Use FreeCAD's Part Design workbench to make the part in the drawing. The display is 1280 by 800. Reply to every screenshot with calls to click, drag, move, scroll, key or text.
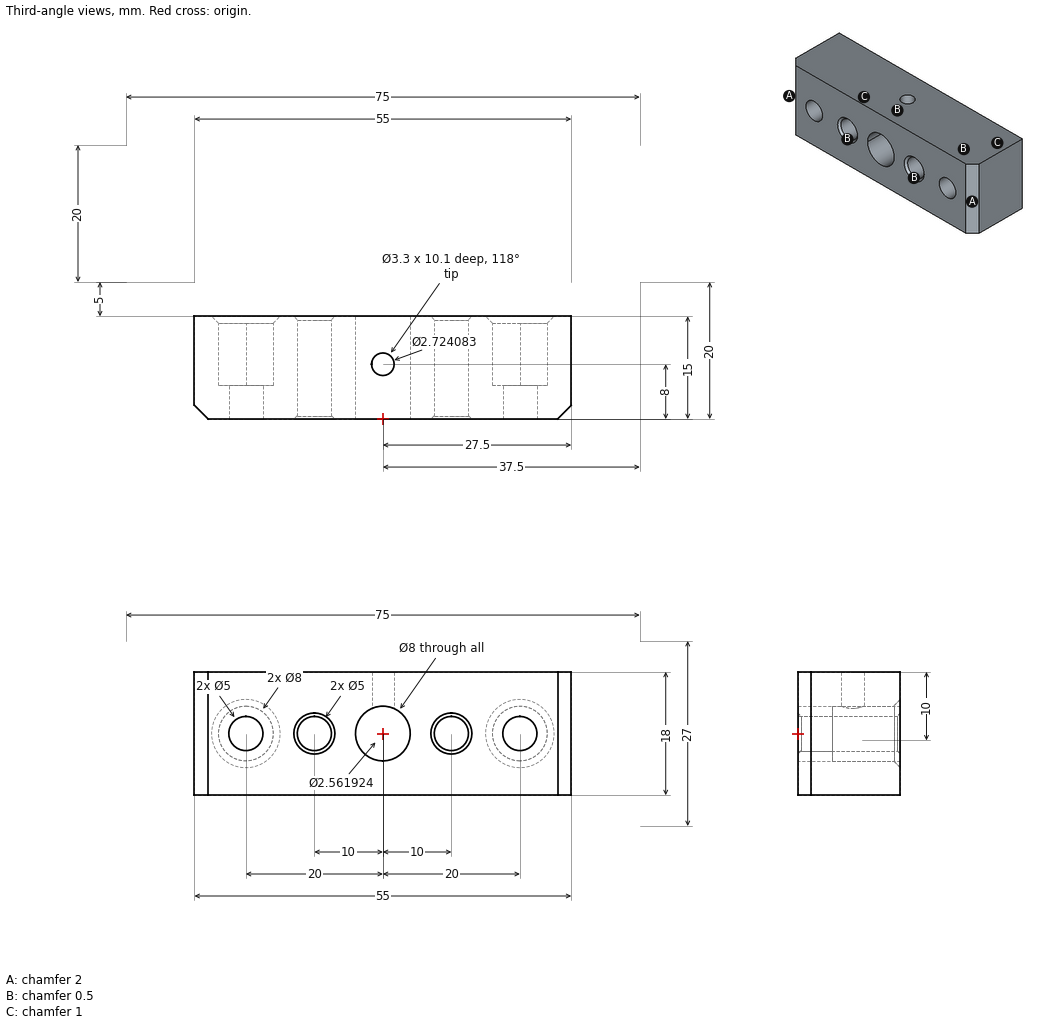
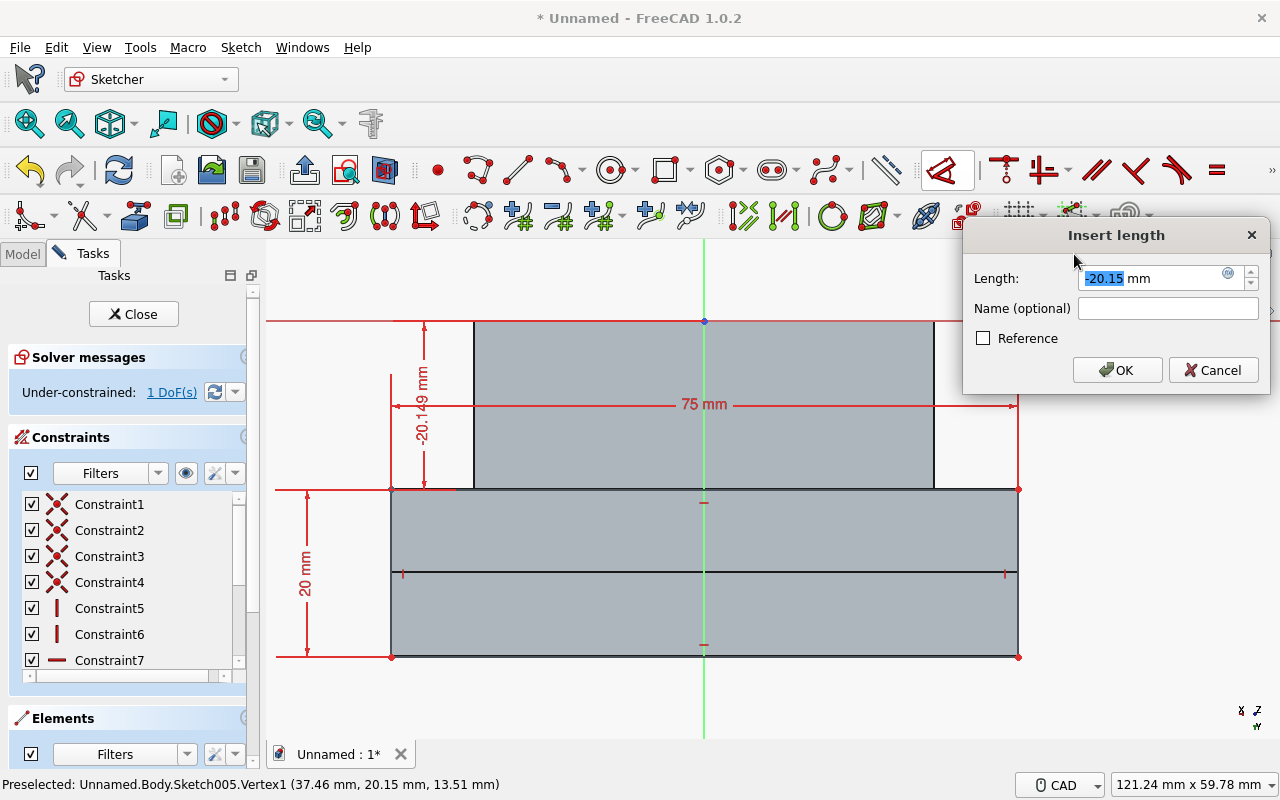
text(-20)
key(Return)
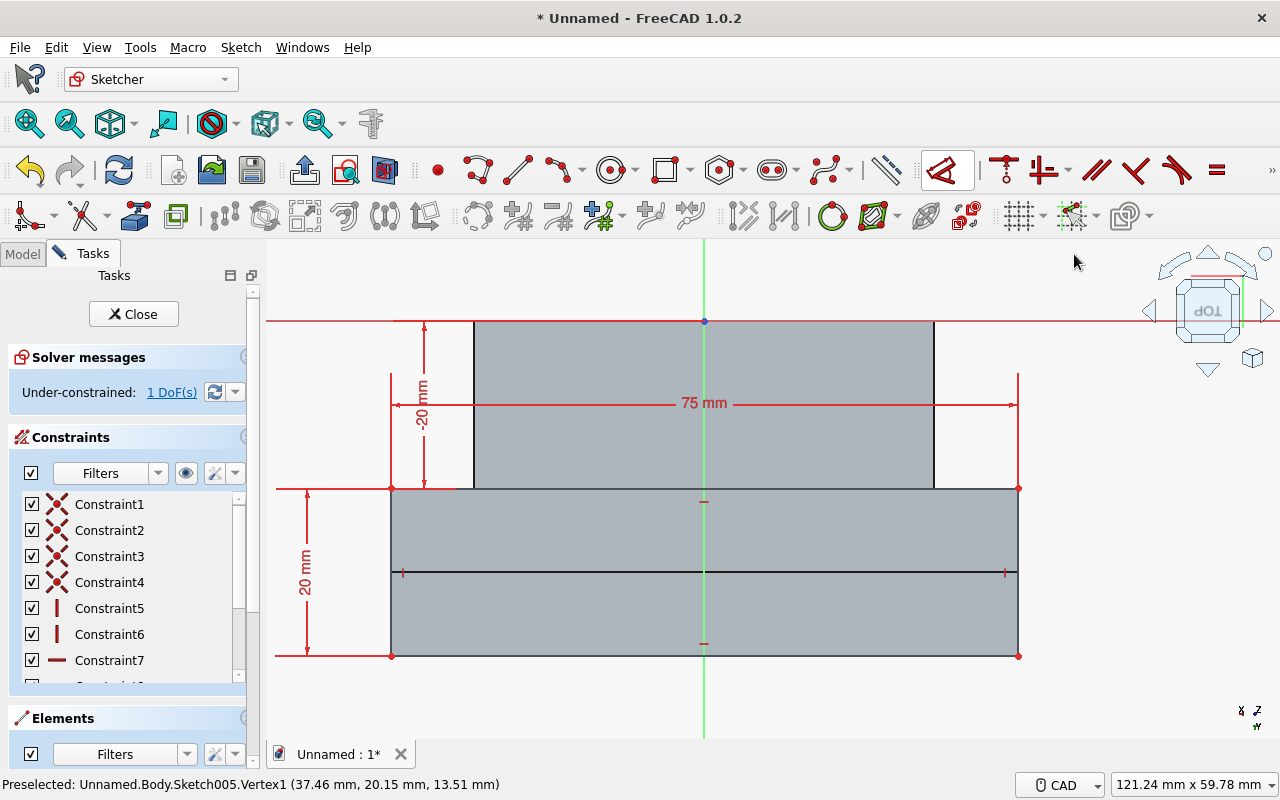
click(391, 489)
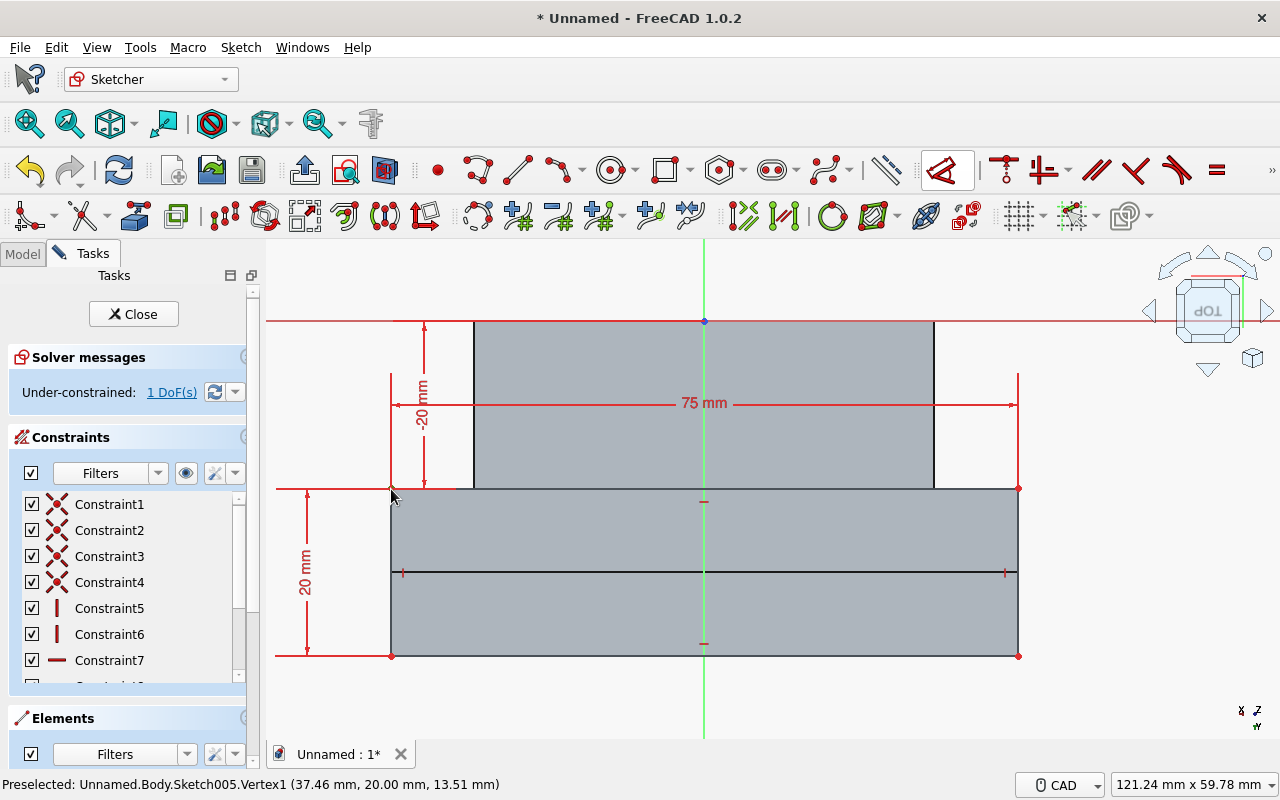
click(968, 170)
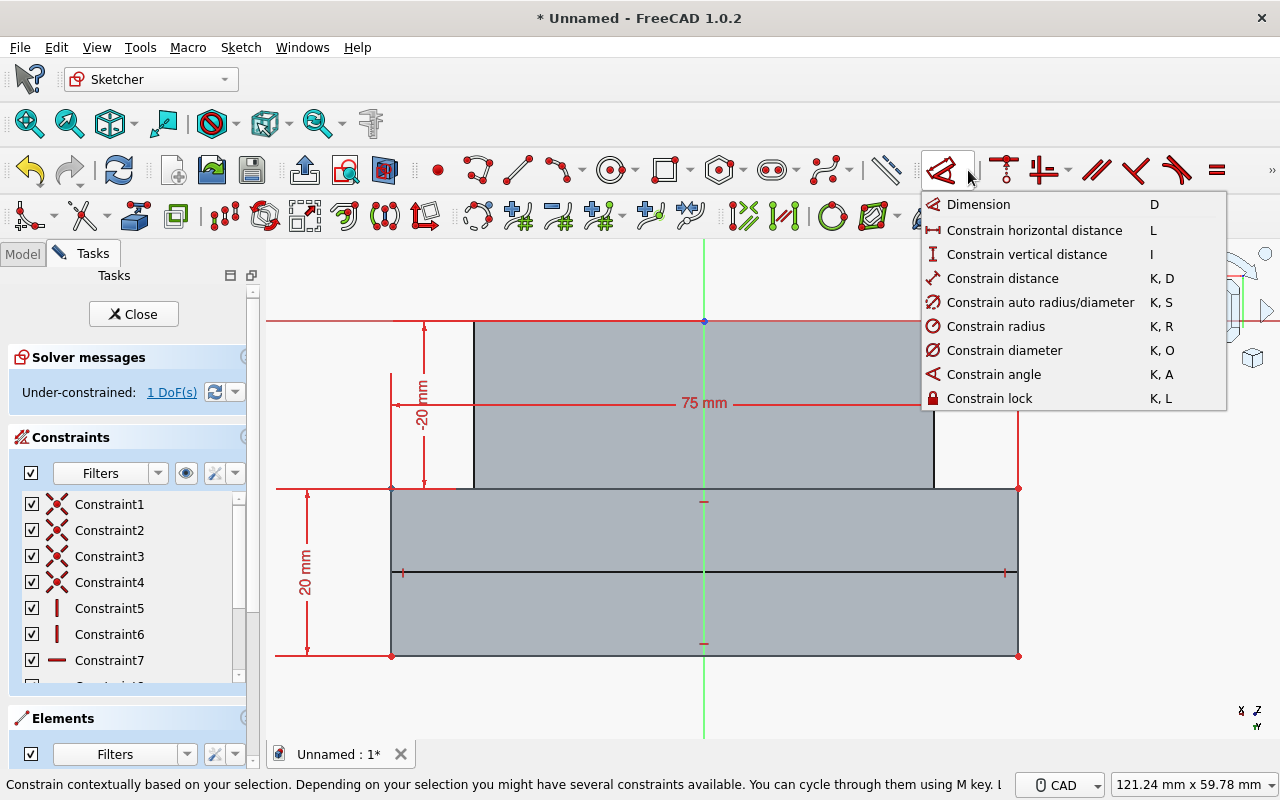
click(1074, 230)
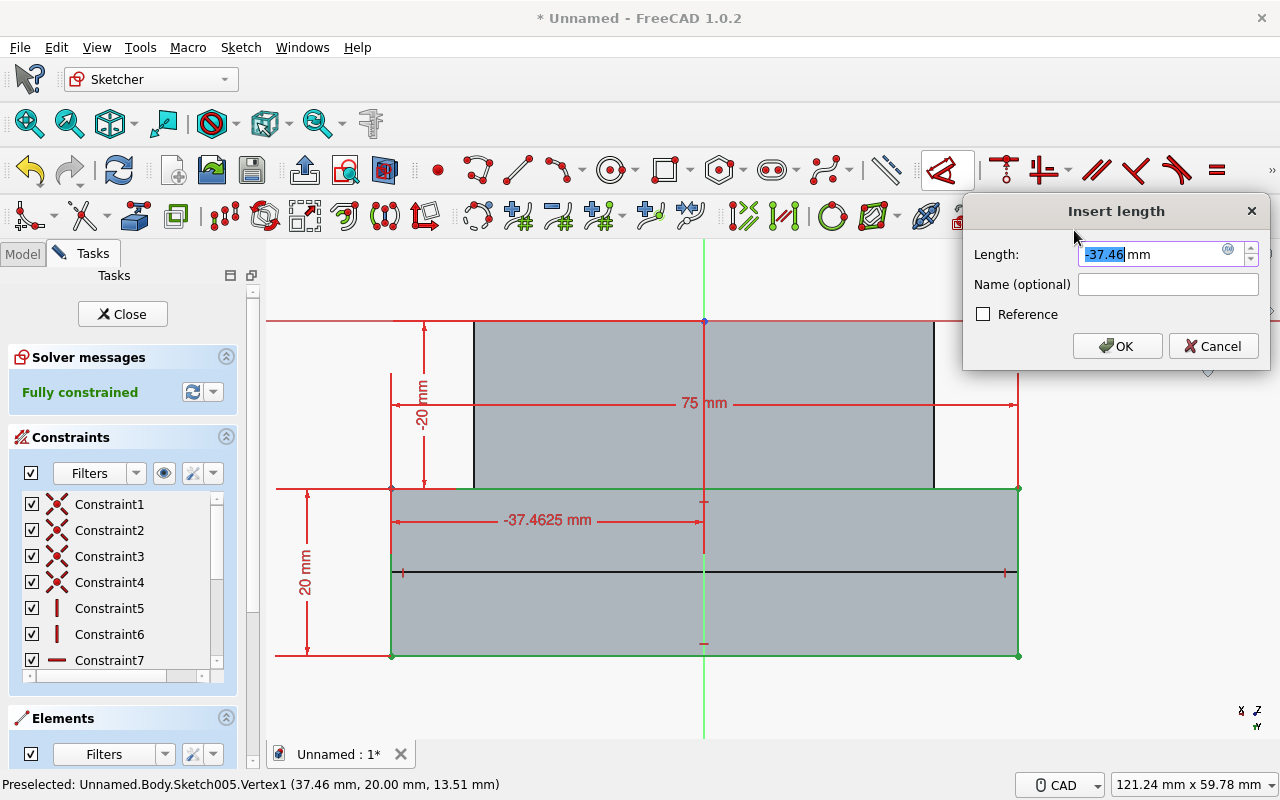
text(-37.5)
key(Return)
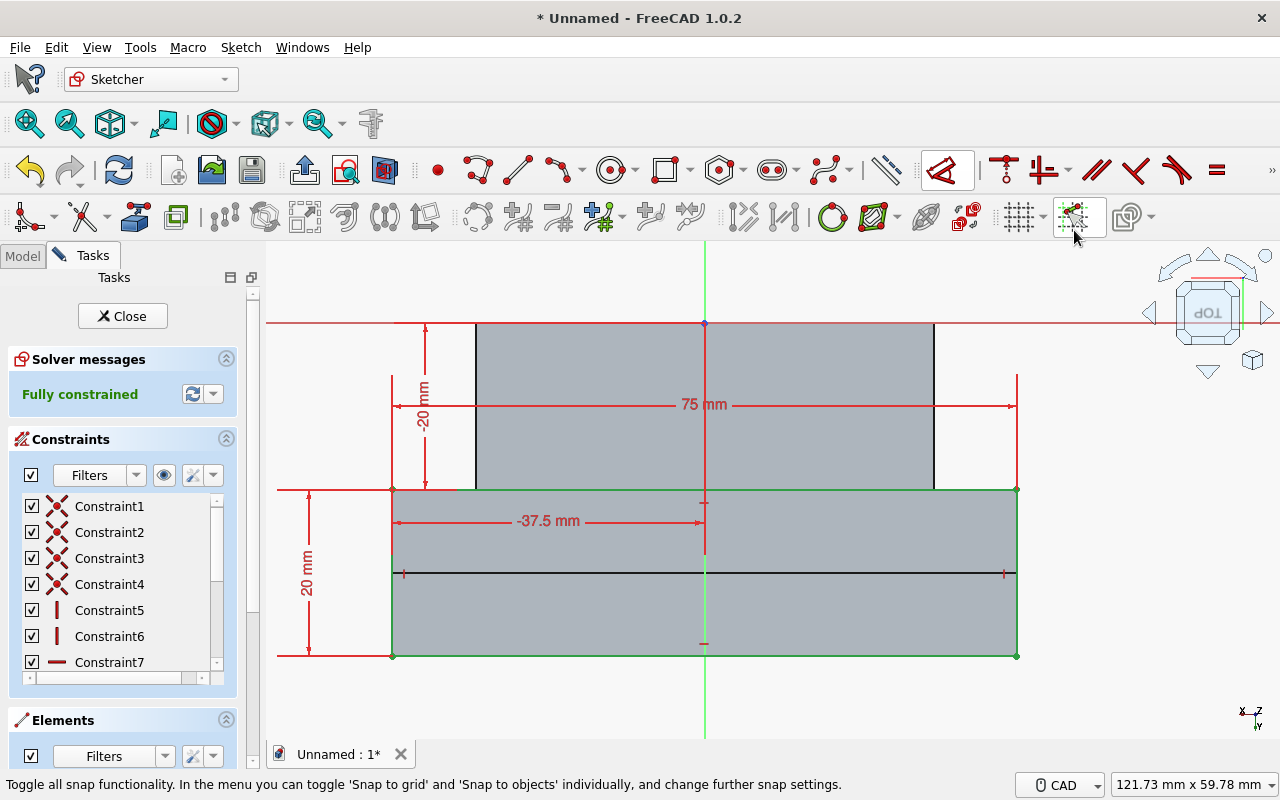
click(123, 316)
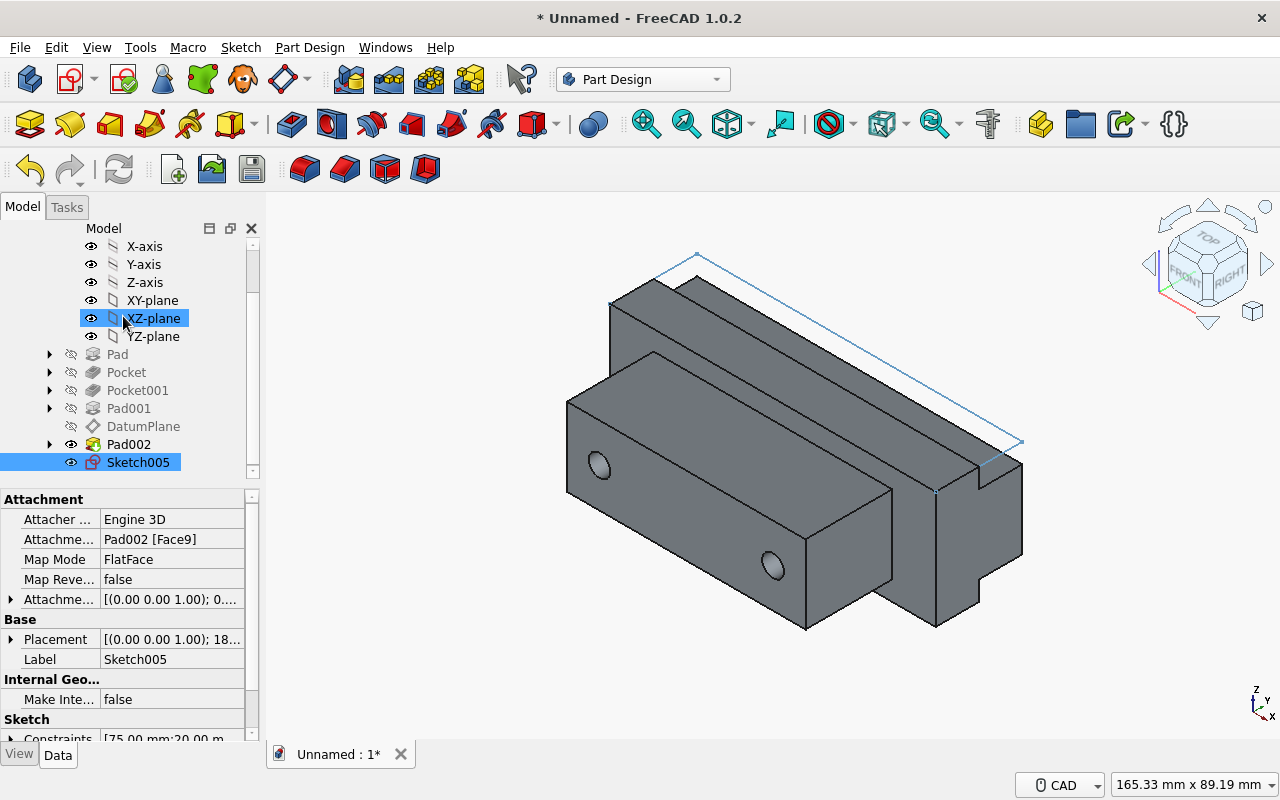
click(292, 124)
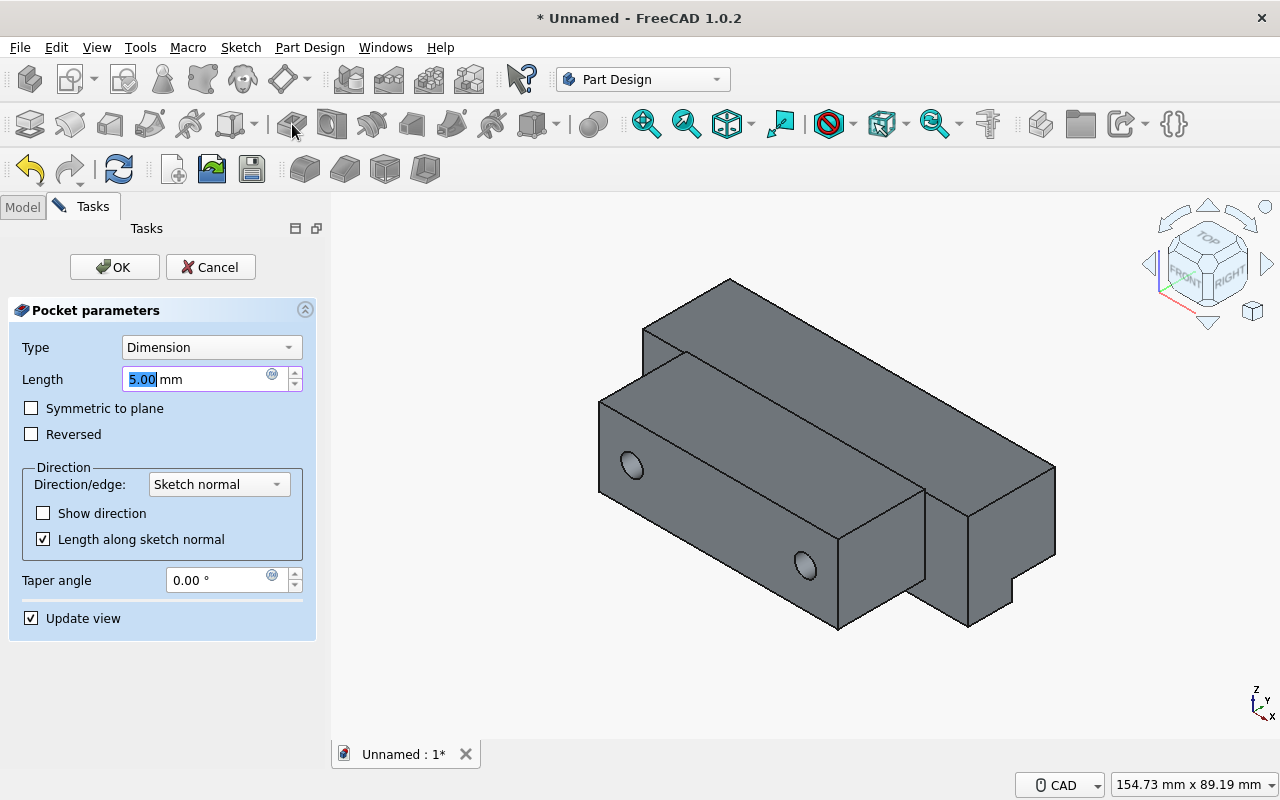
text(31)
key(Tab)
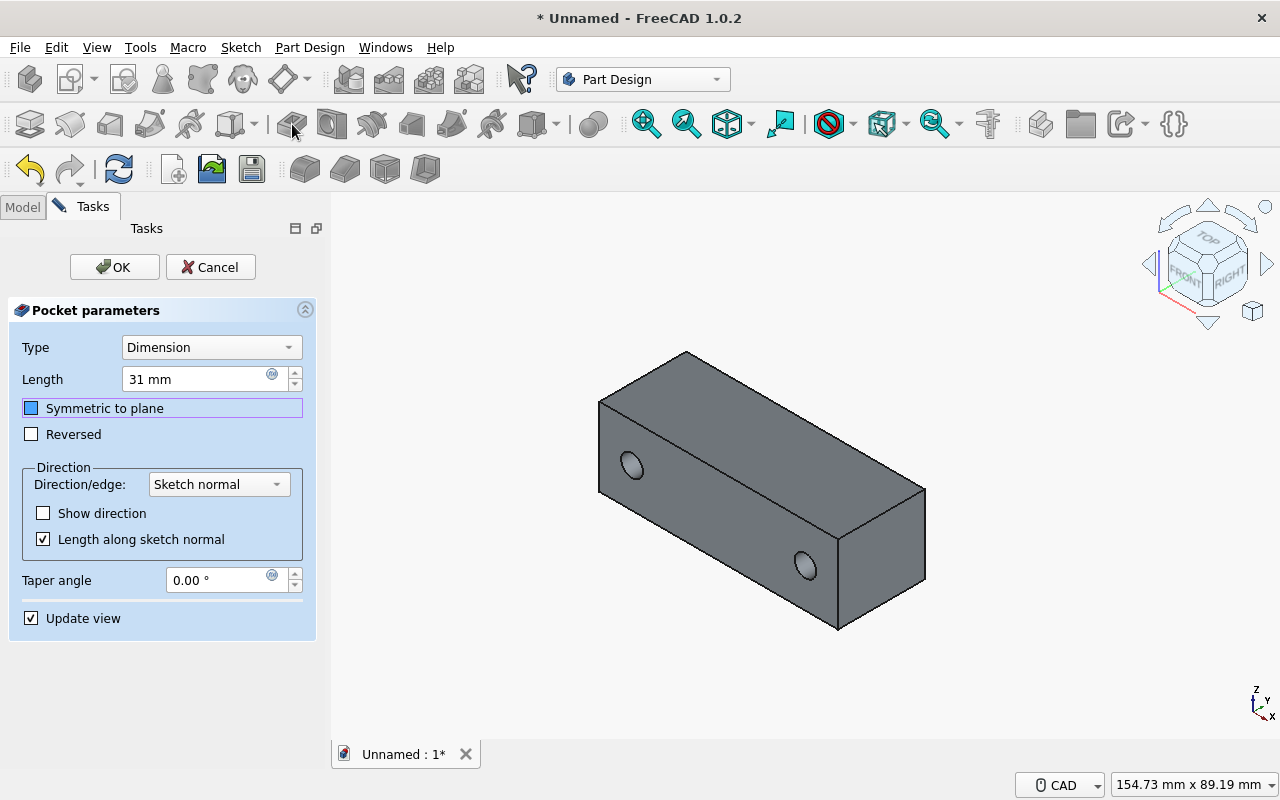
click(115, 267)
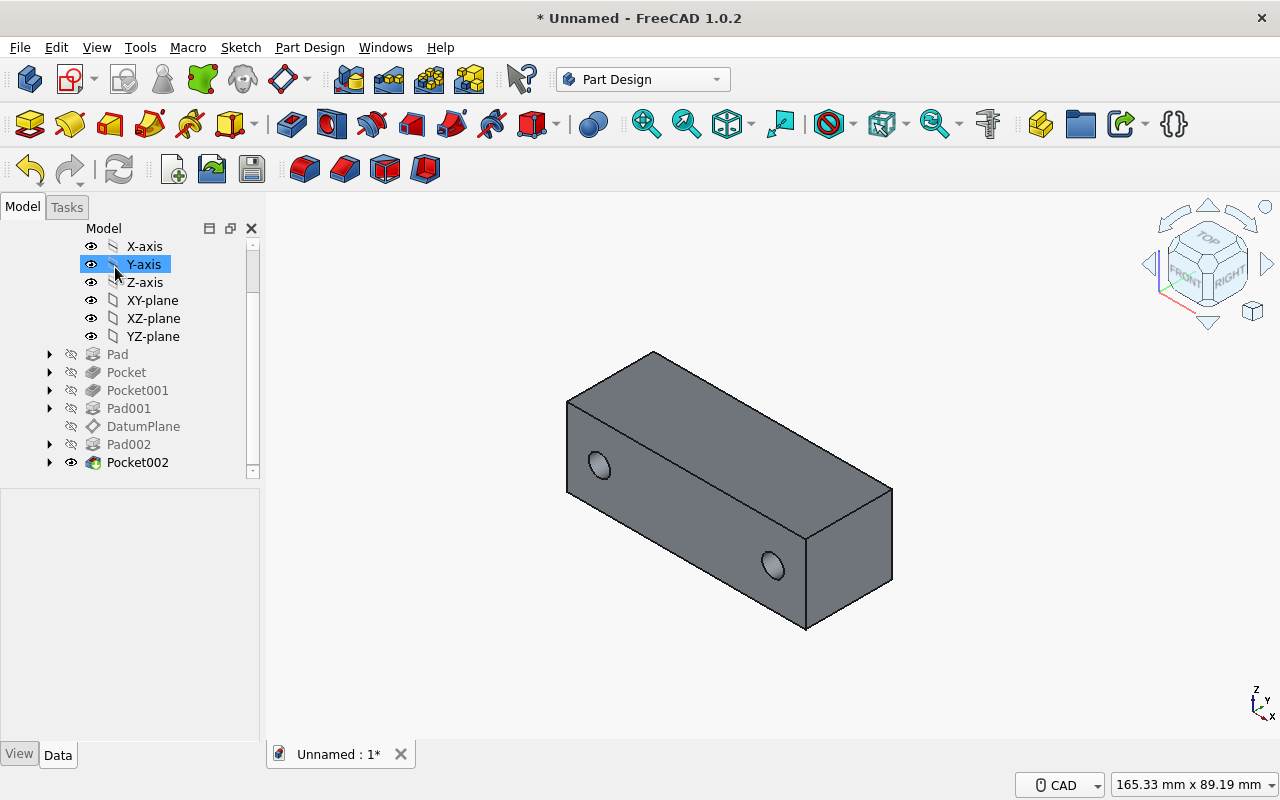
key(4)